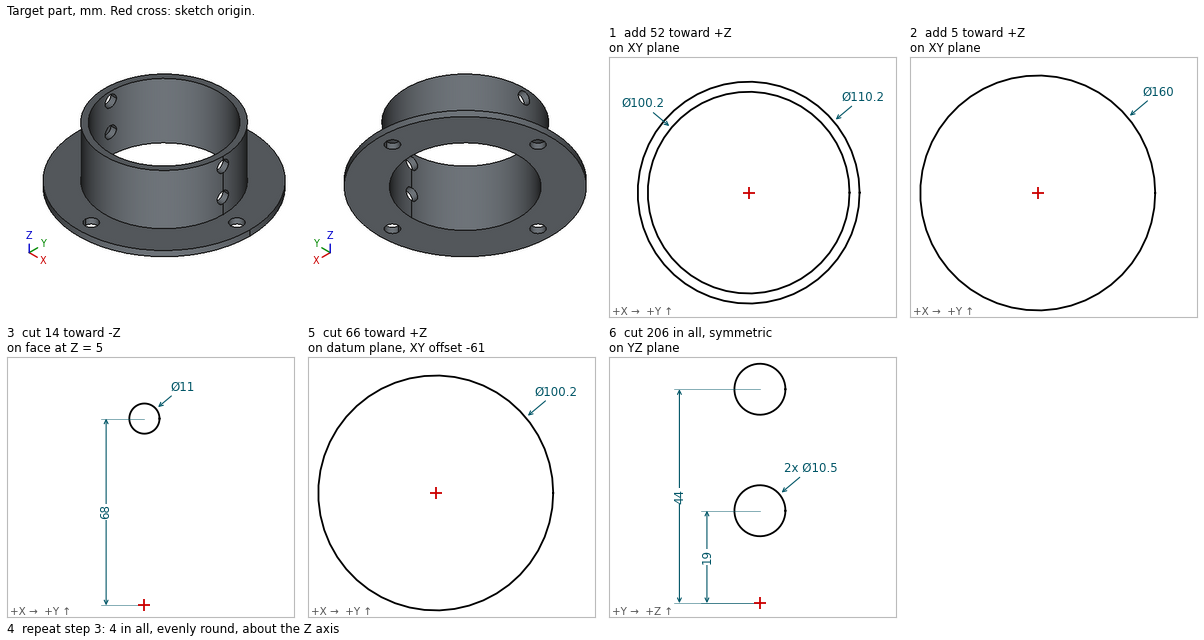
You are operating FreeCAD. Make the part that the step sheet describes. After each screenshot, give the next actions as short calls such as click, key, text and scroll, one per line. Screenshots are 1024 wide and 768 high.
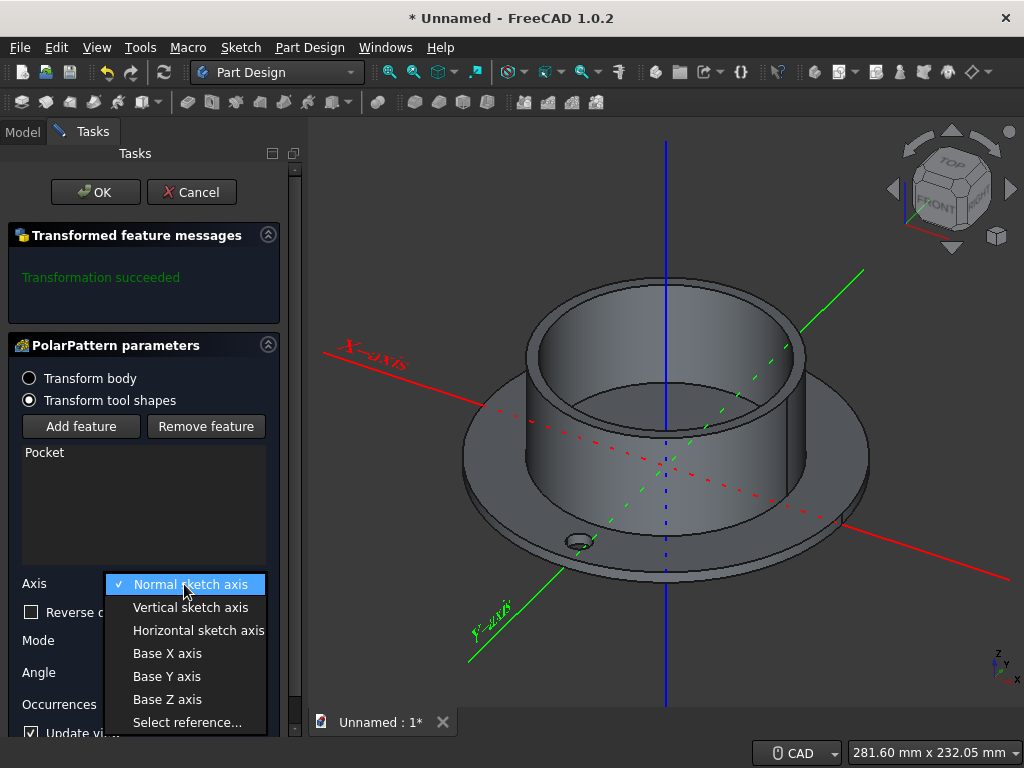
click(184, 700)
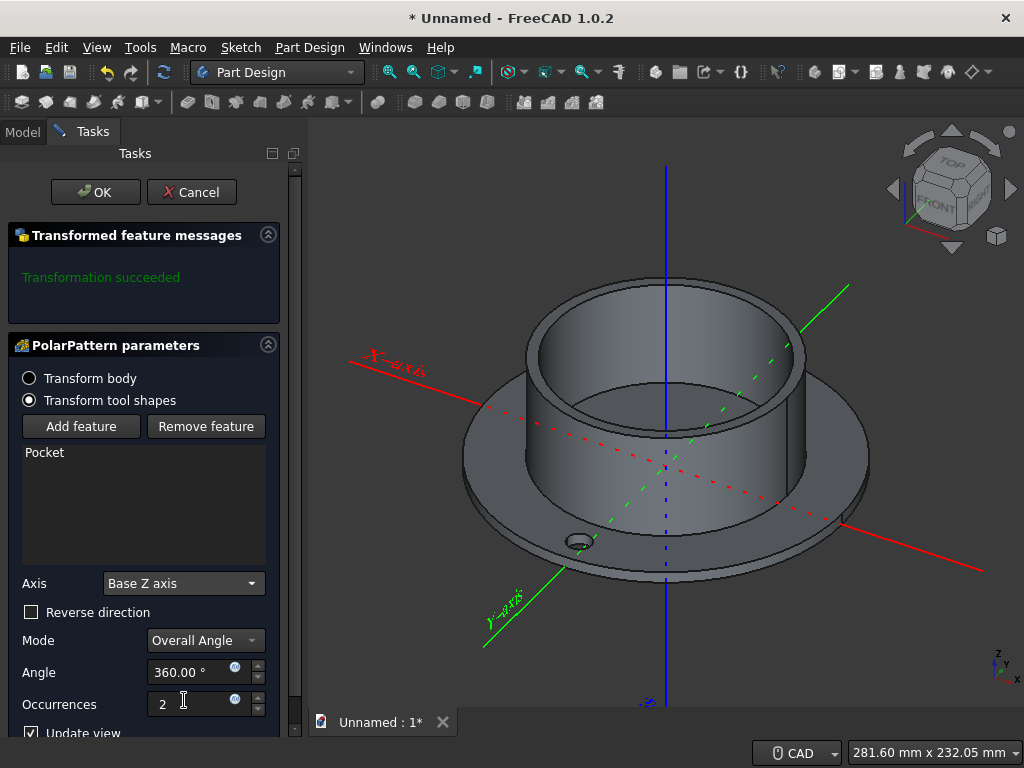
triple_click(198, 704)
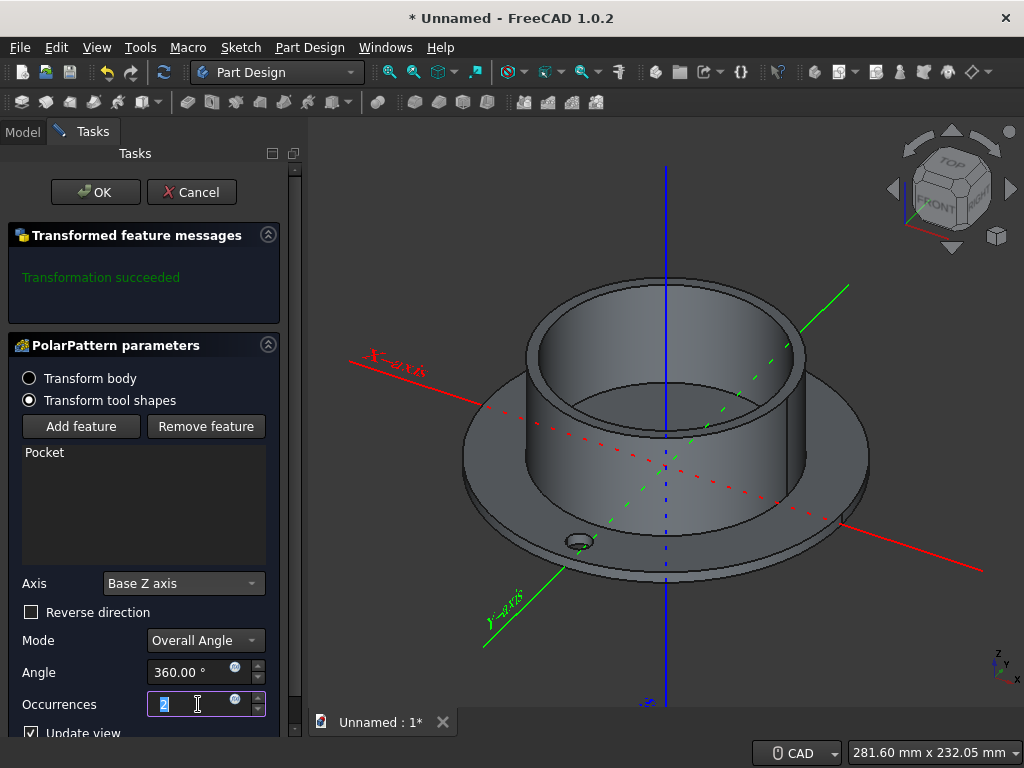
text(4)
key(Tab)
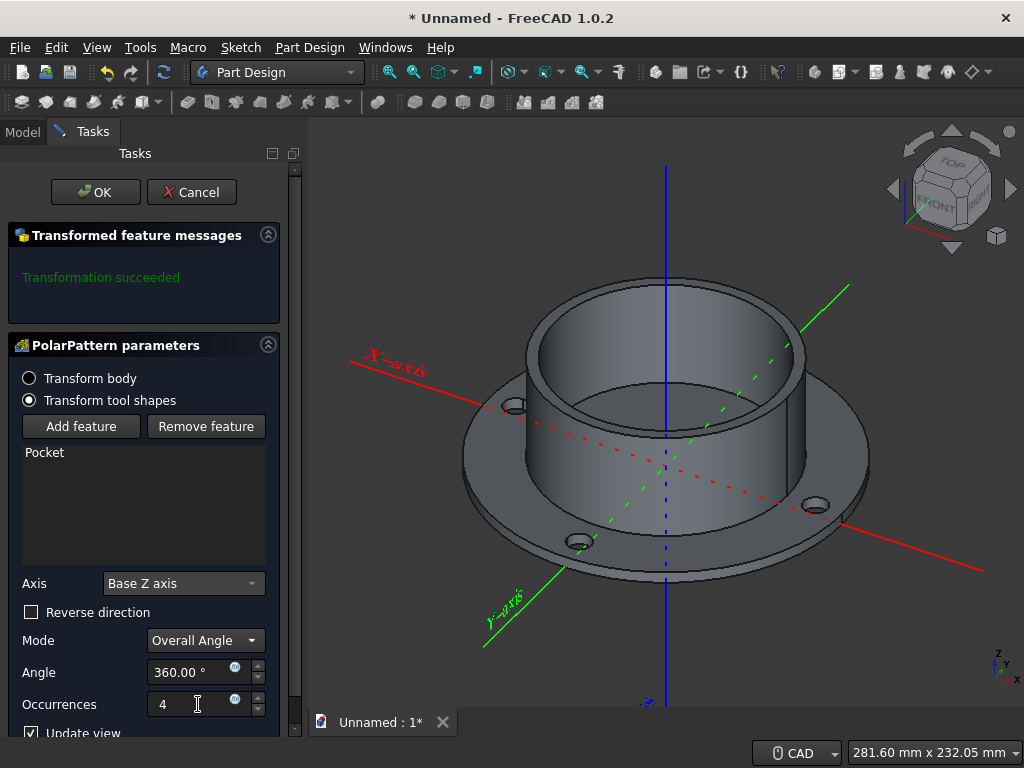
click(96, 192)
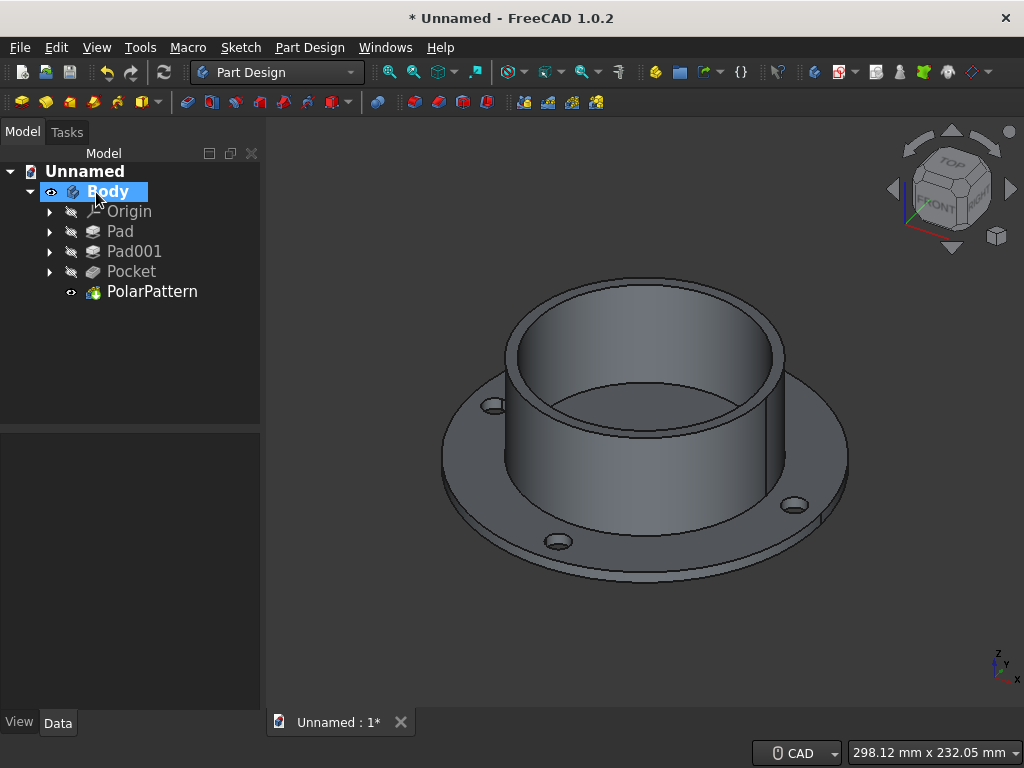
click(50, 212)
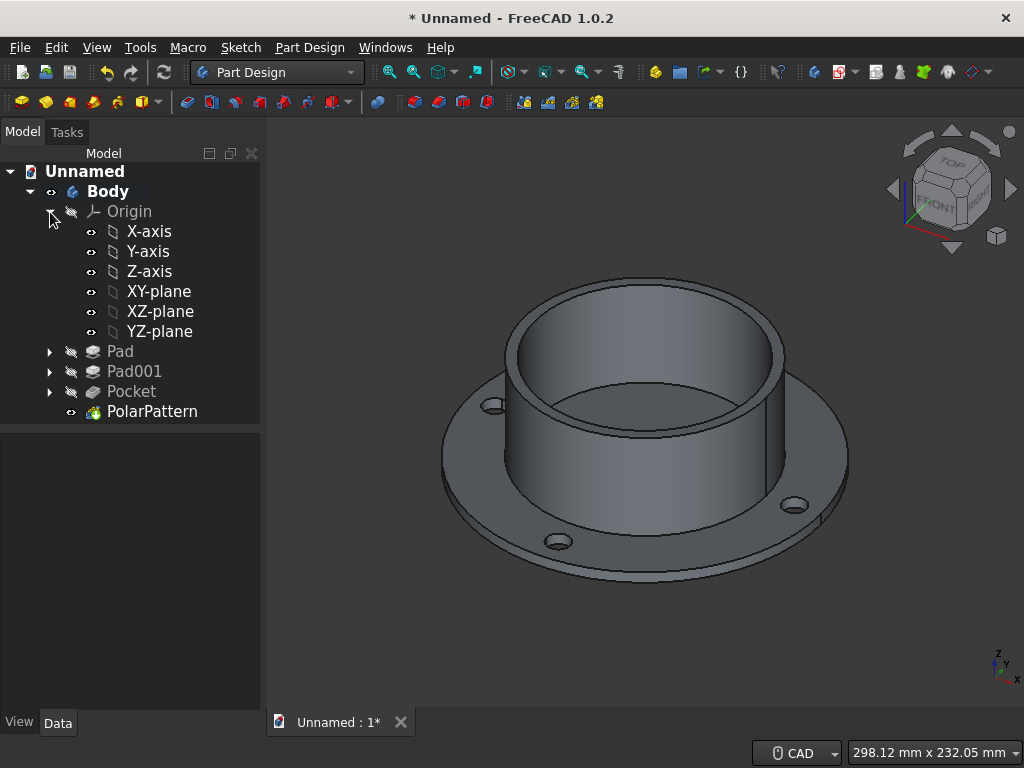
click(136, 292)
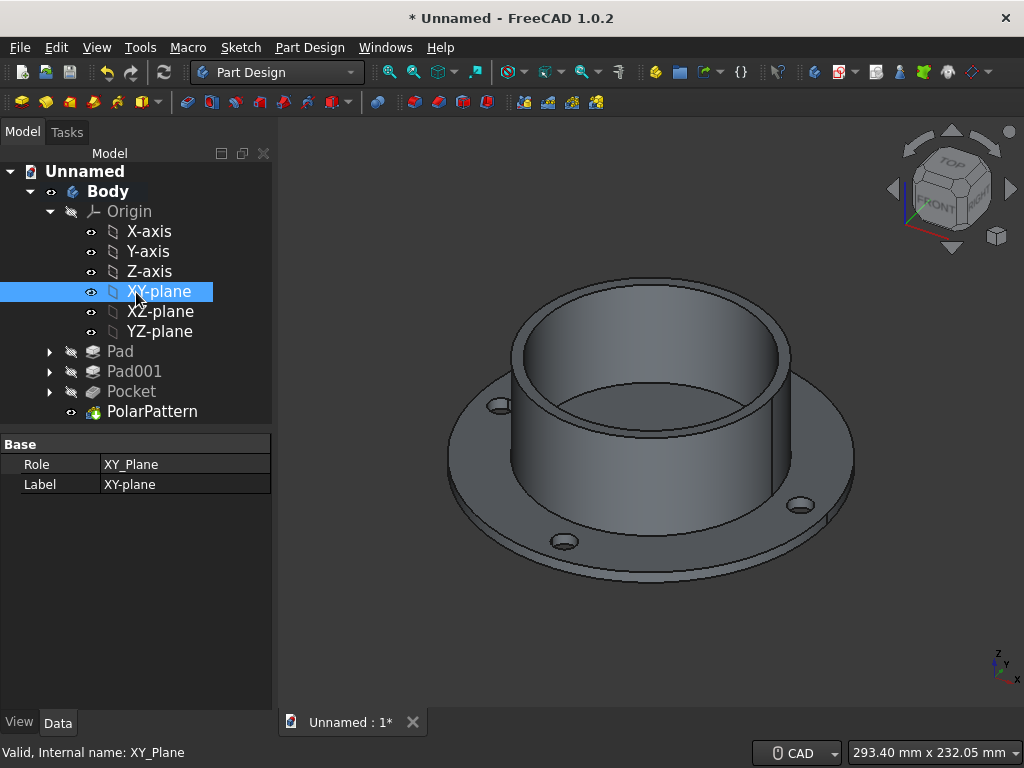
click(972, 72)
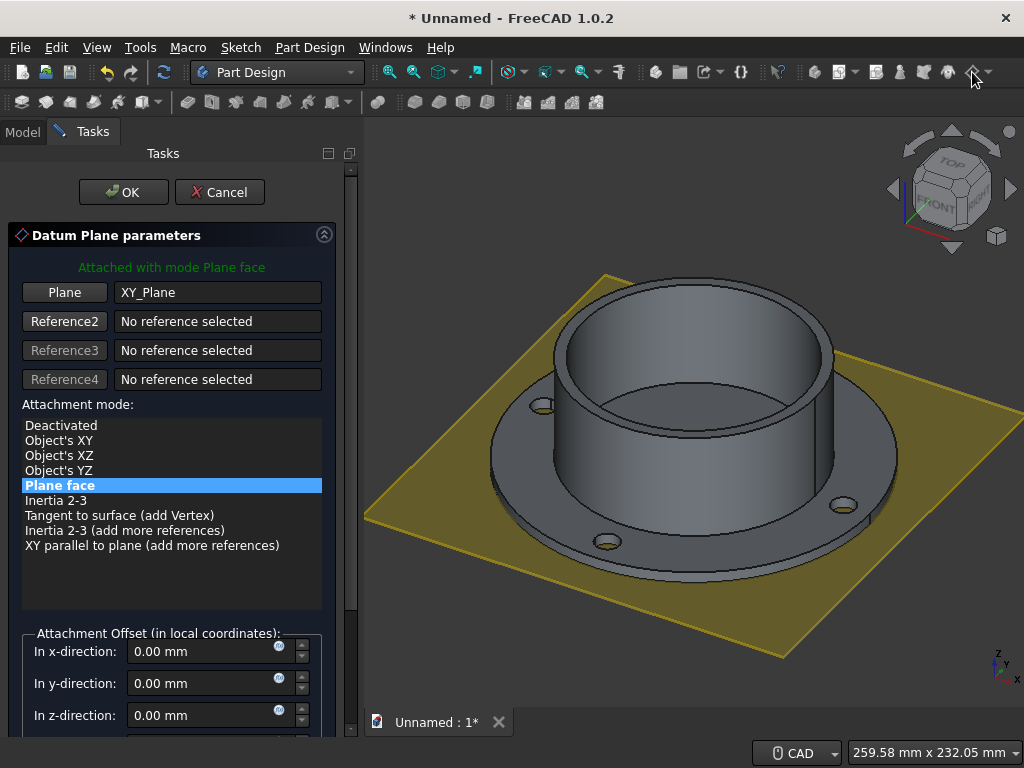
triple_click(210, 715)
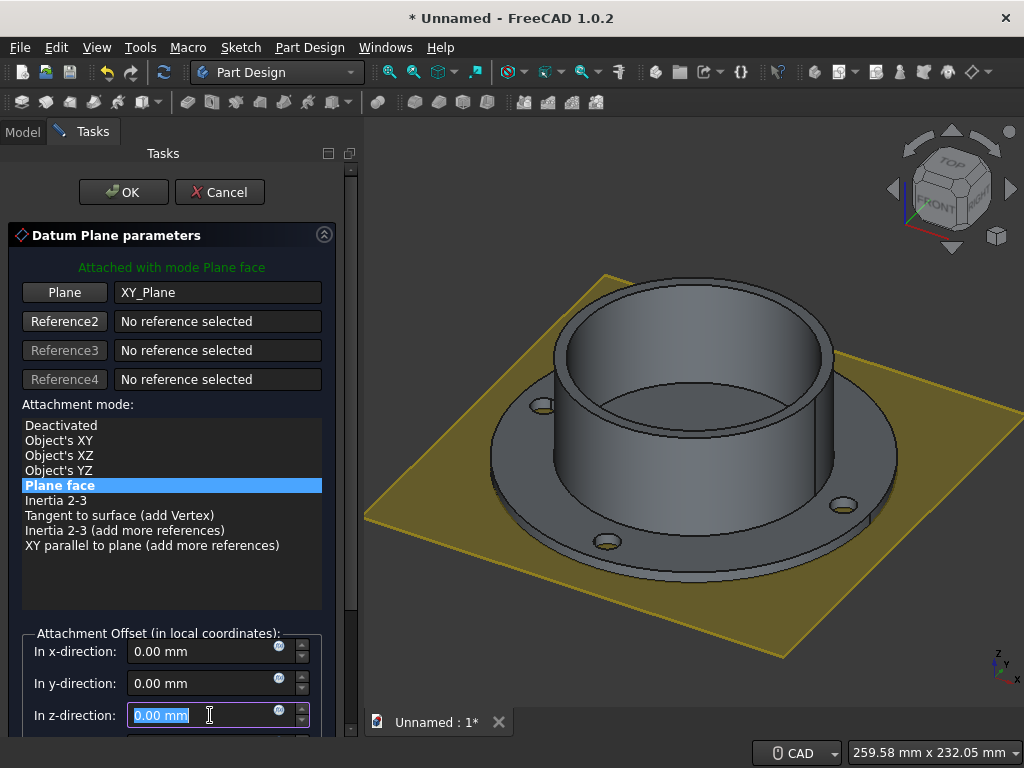
text(-61)
key(Tab)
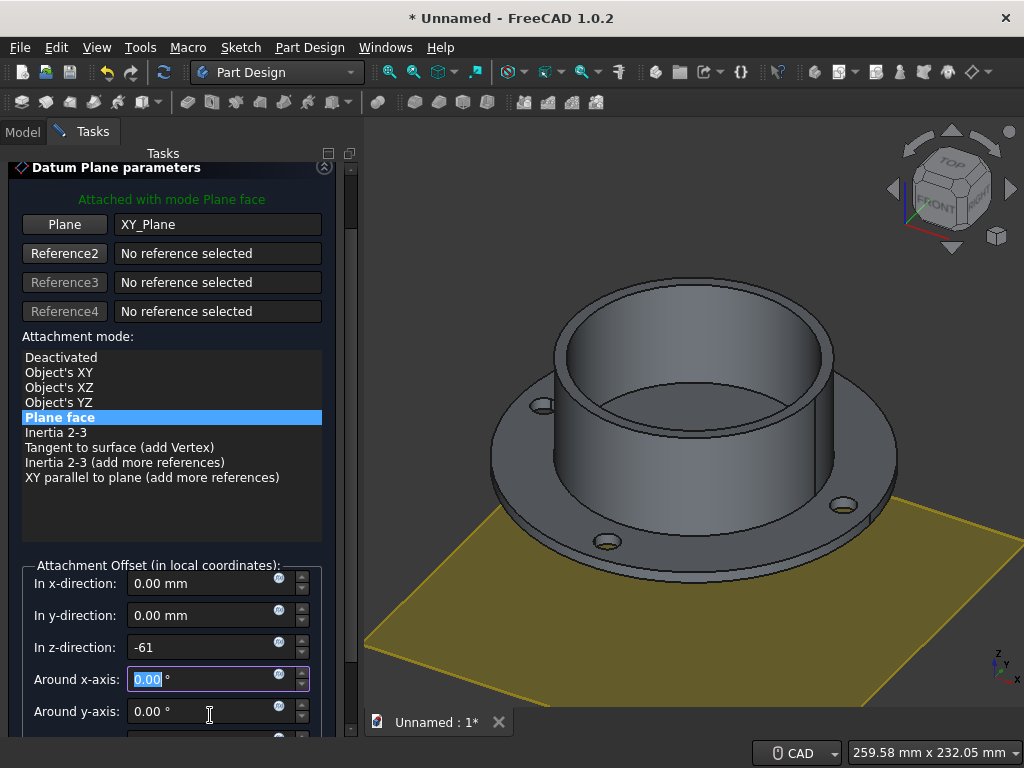
scroll(351, 450, up, 2)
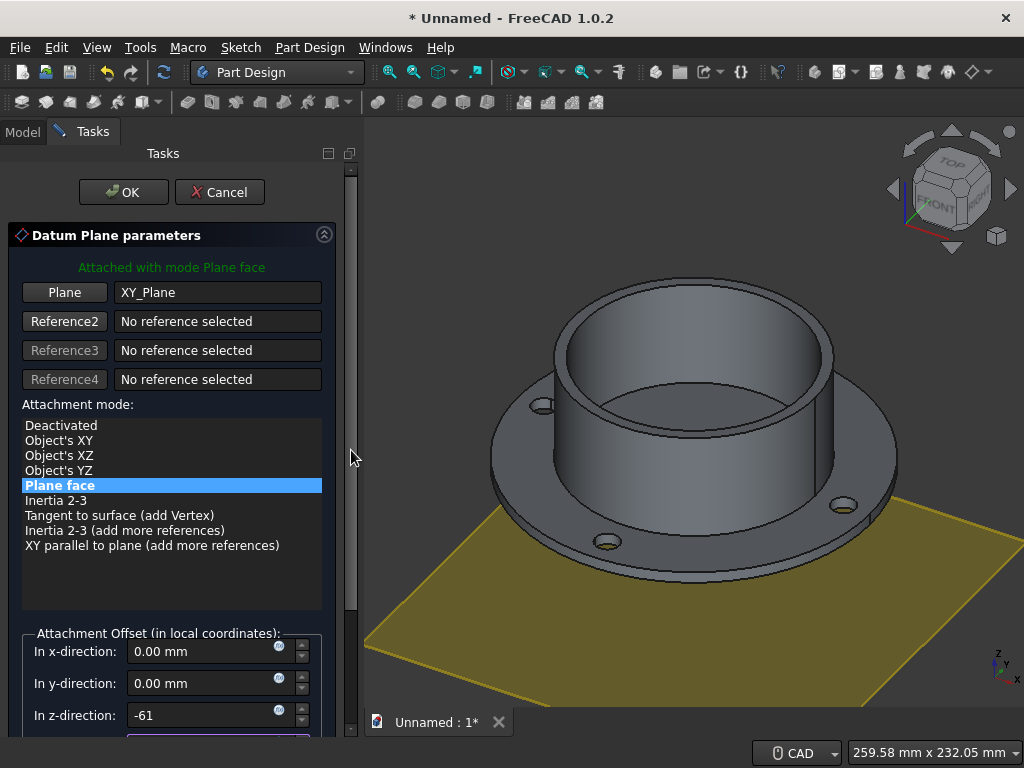
click(124, 192)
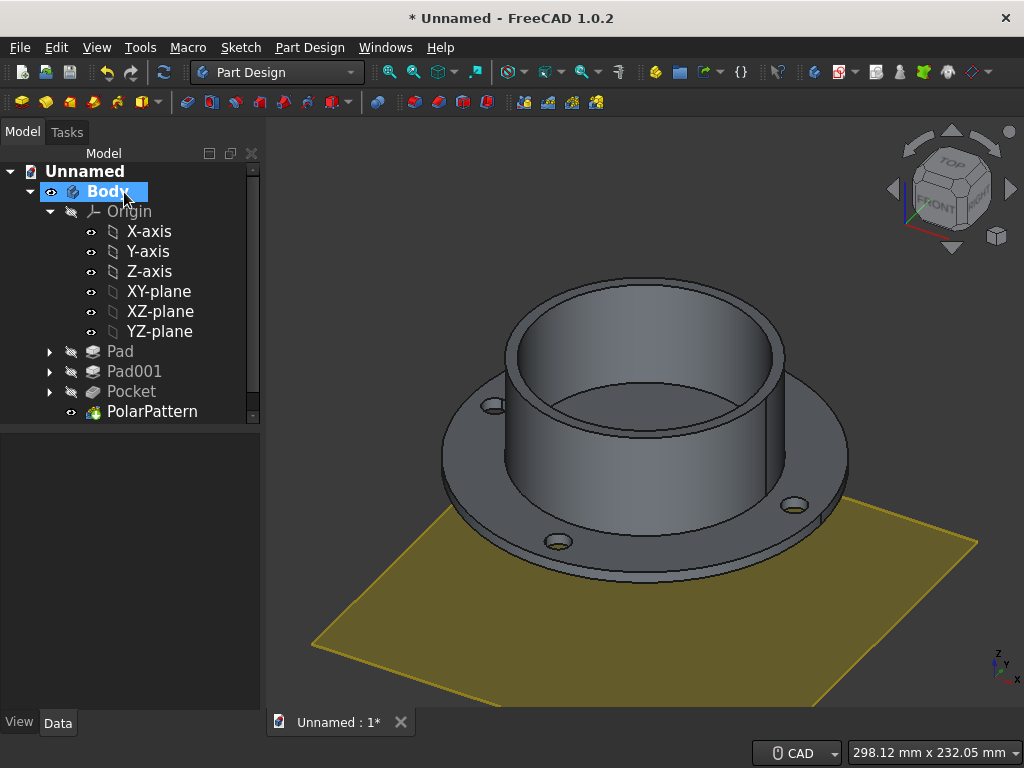
scroll(100, 287, down, 3)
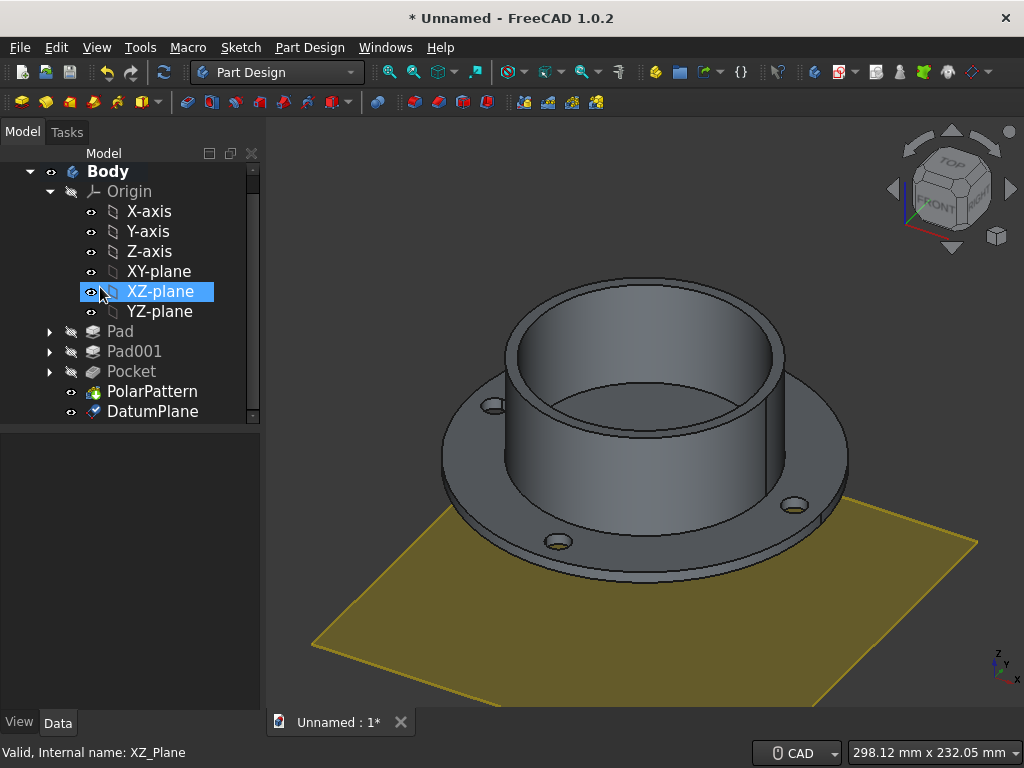
click(116, 412)